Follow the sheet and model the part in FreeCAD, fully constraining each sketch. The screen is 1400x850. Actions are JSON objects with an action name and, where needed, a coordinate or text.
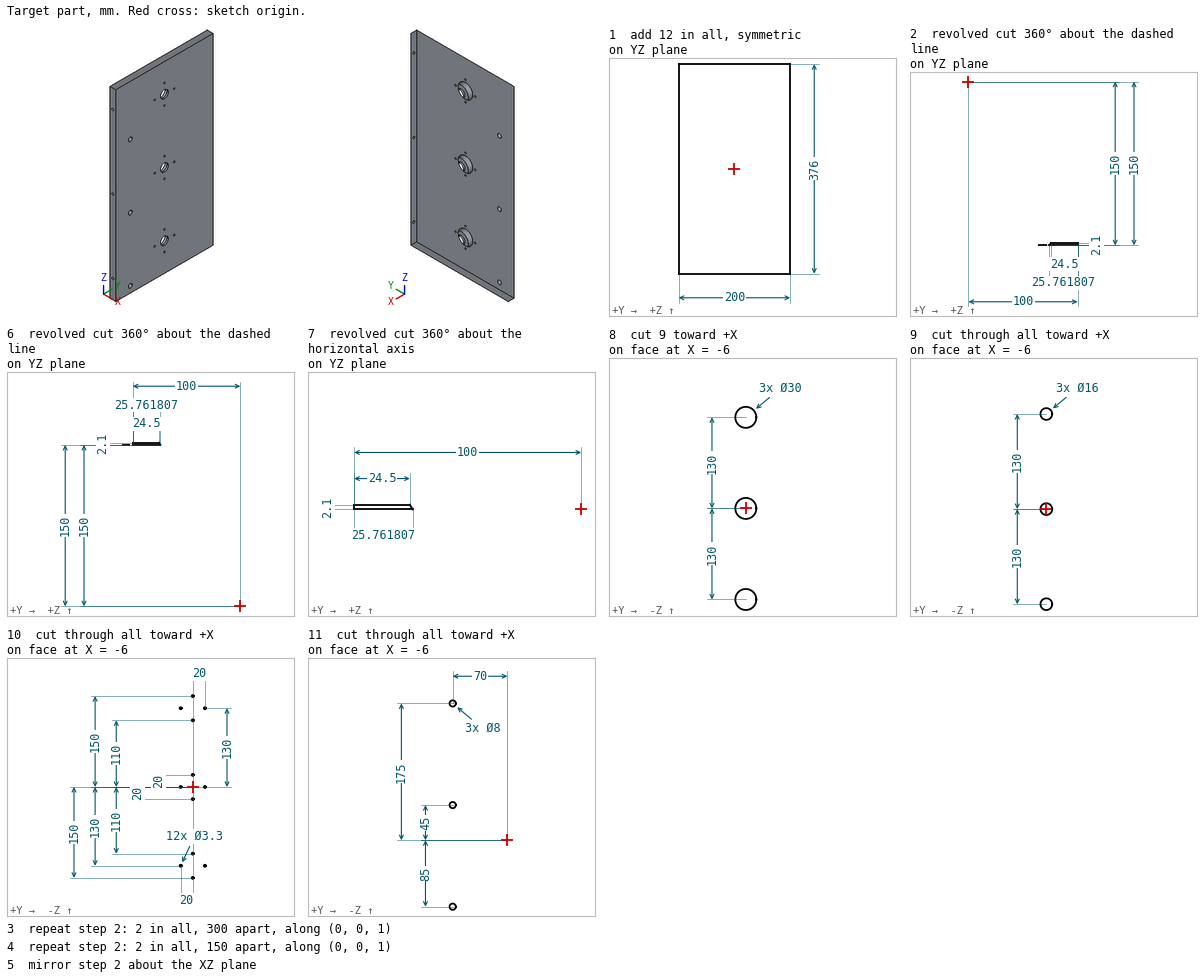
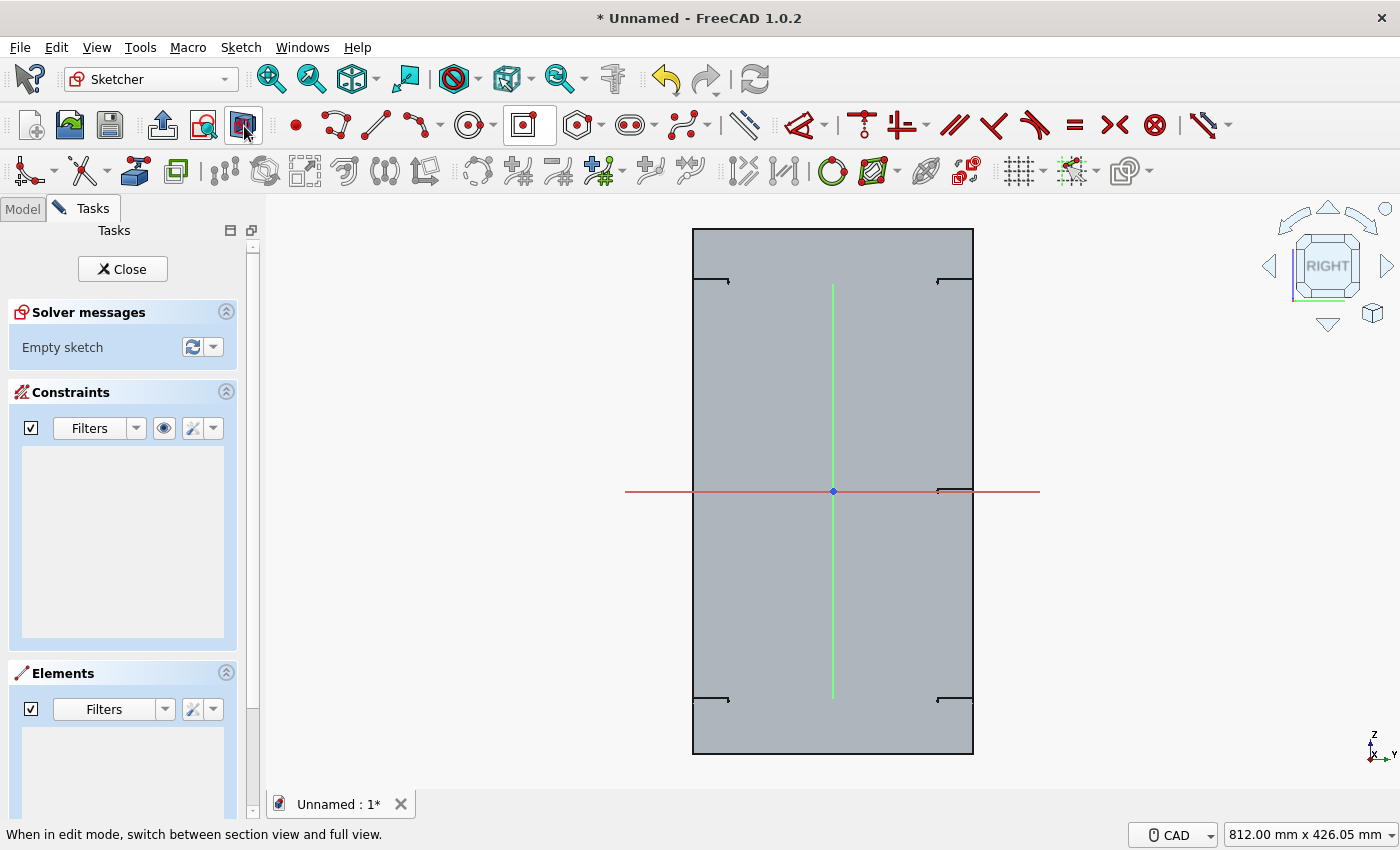
{"action": "scroll", "coordinate": [709, 490], "scroll_direction": "up", "scroll_amount": 15}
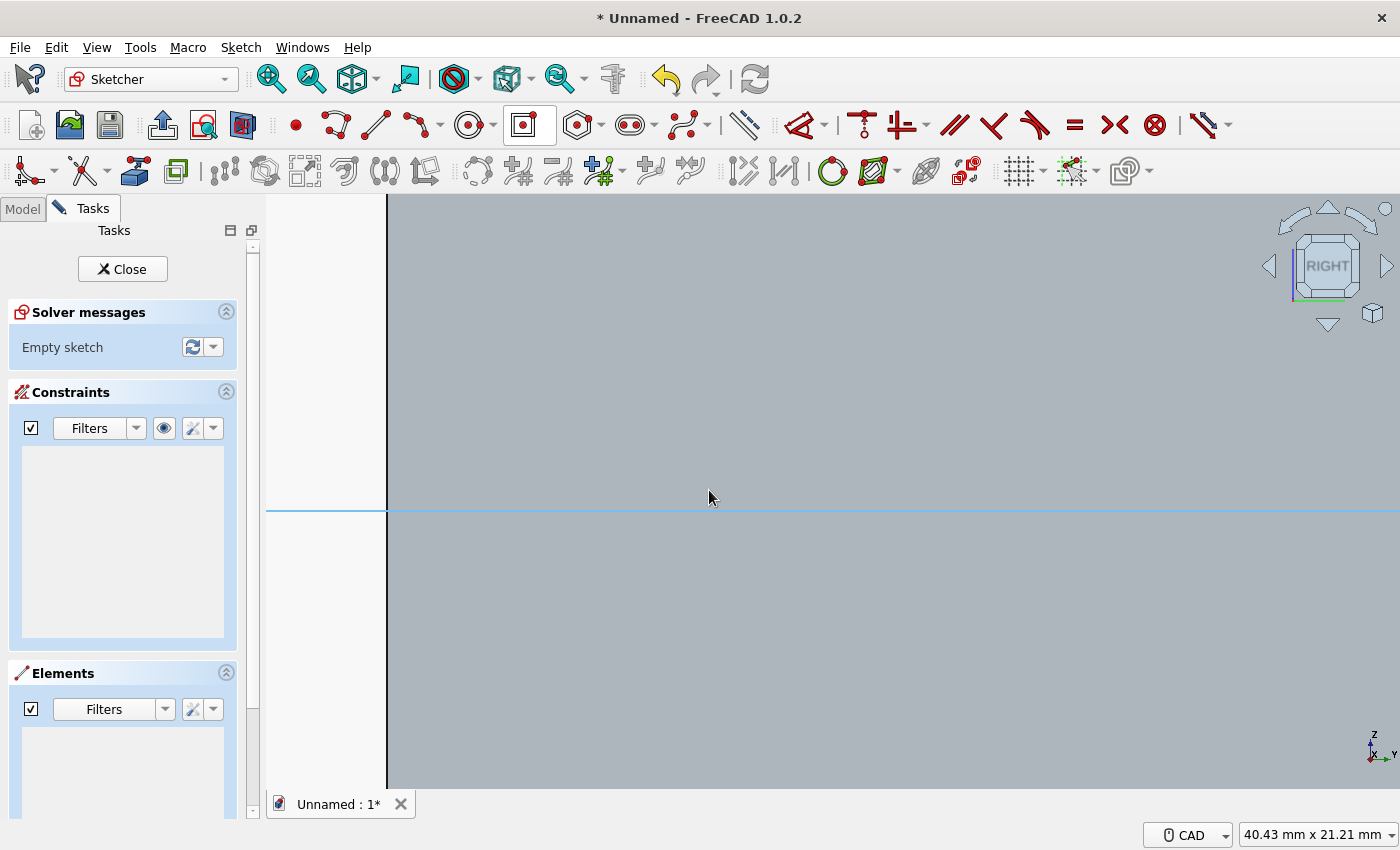
{"action": "left_click", "coordinate": [336, 126]}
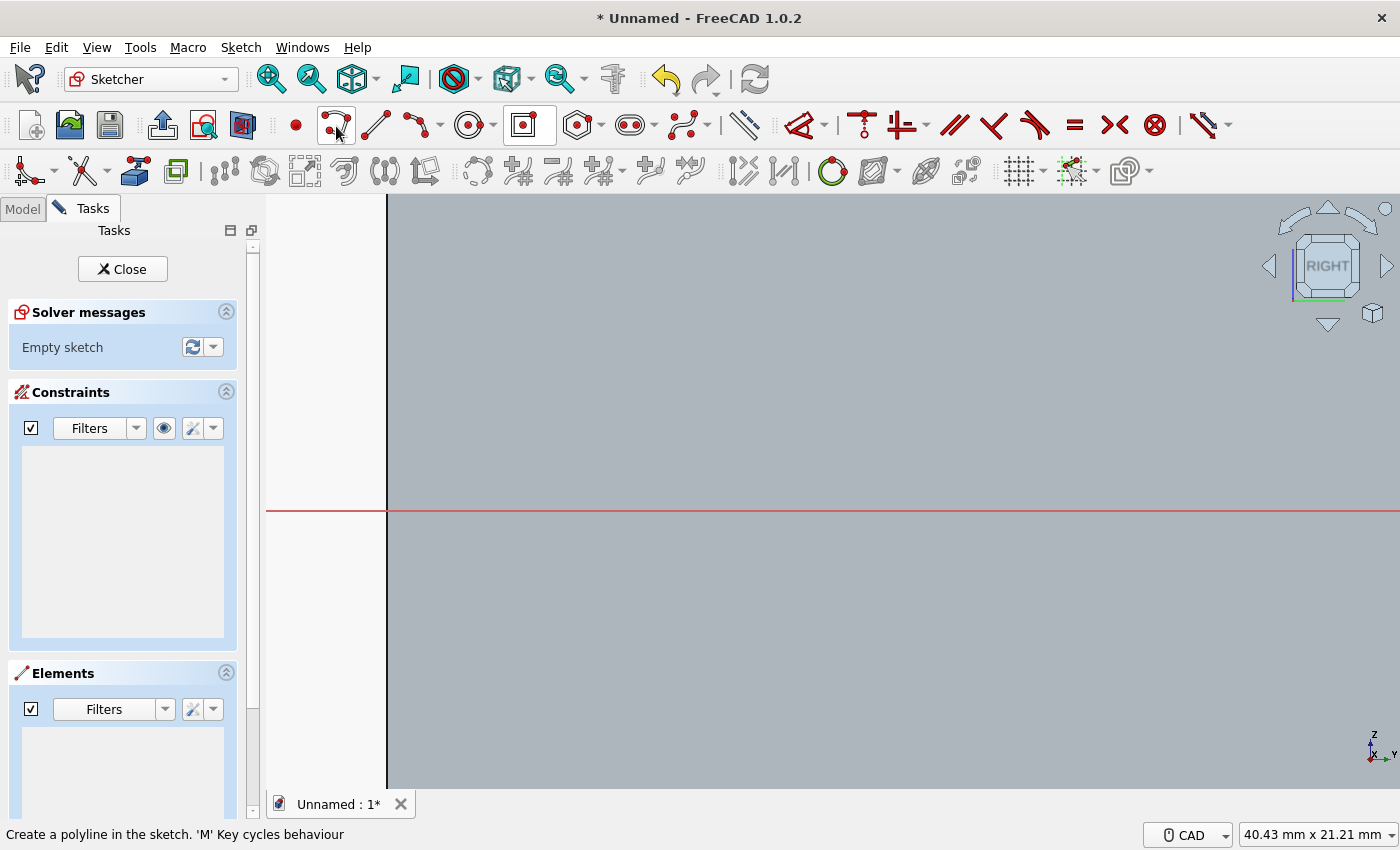
{"action": "left_click", "coordinate": [1110, 511]}
{"action": "left_click", "coordinate": [1074, 452]}
{"action": "left_click", "coordinate": [387, 452]}
{"action": "left_click", "coordinate": [387, 502]}
{"action": "left_click", "coordinate": [1110, 511]}
{"action": "key", "text": "Escape"}
{"action": "key", "text": "Escape"}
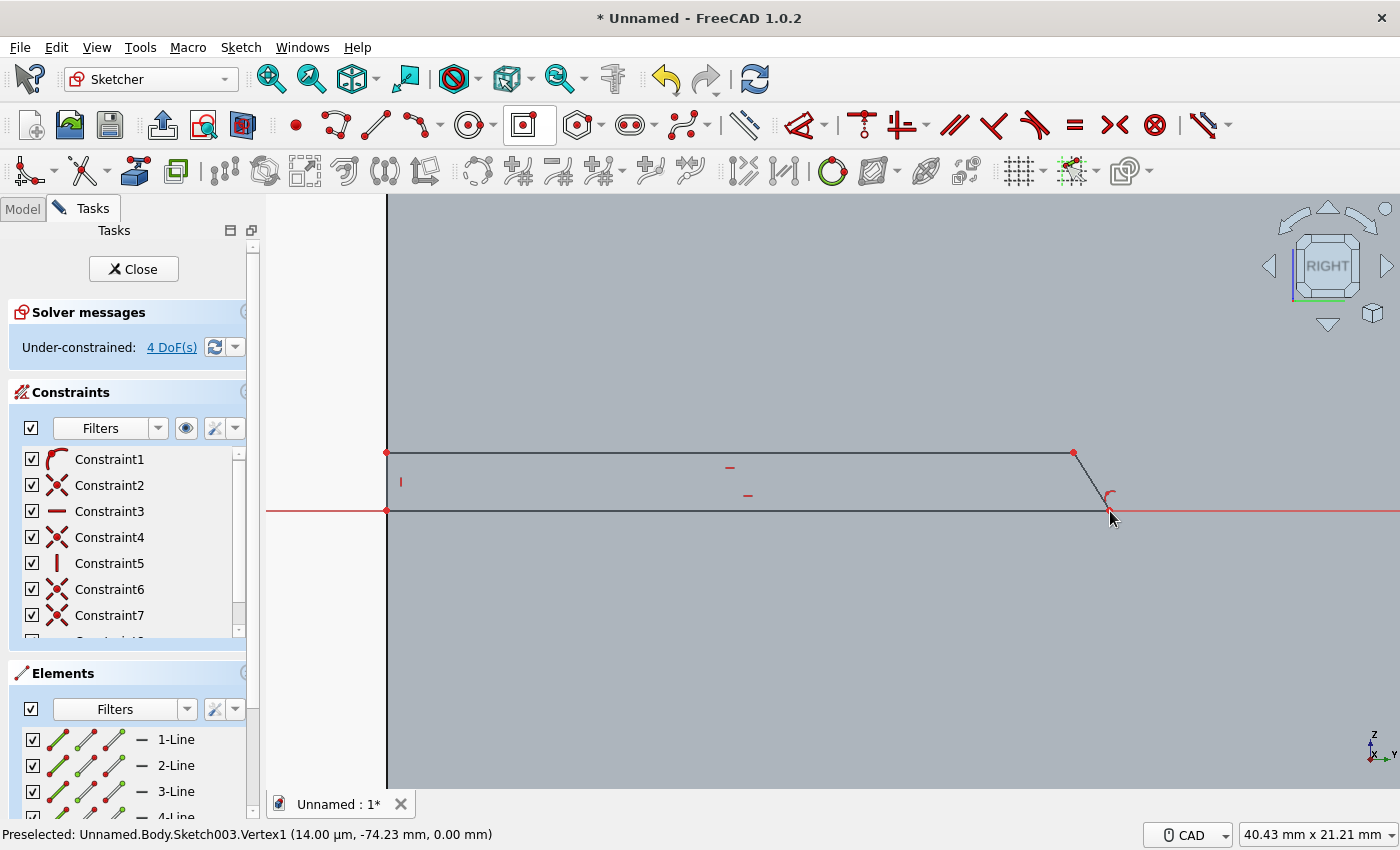
{"action": "left_click", "coordinate": [800, 126]}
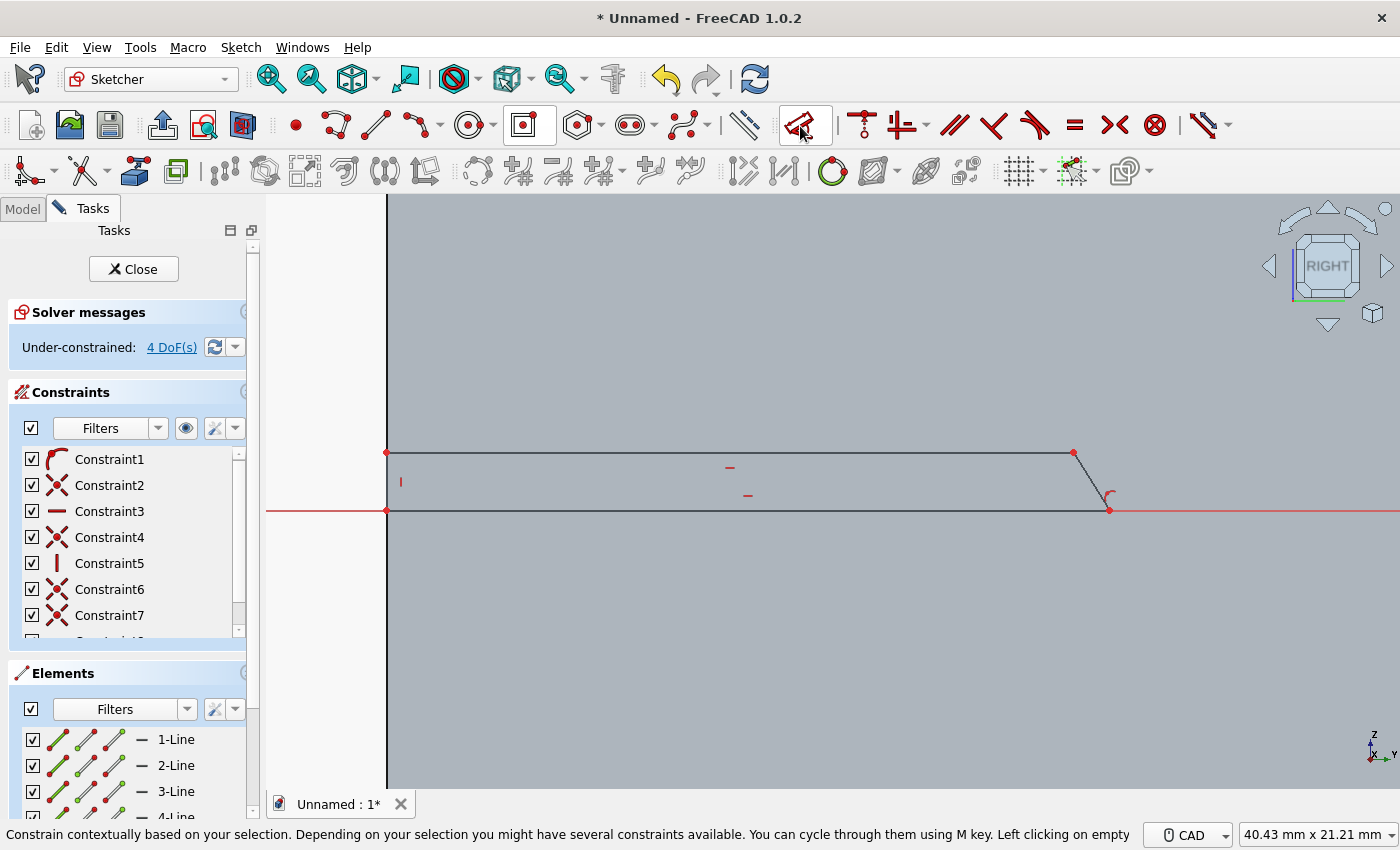
{"action": "left_click", "coordinate": [387, 470]}
{"action": "left_click", "coordinate": [353, 482]}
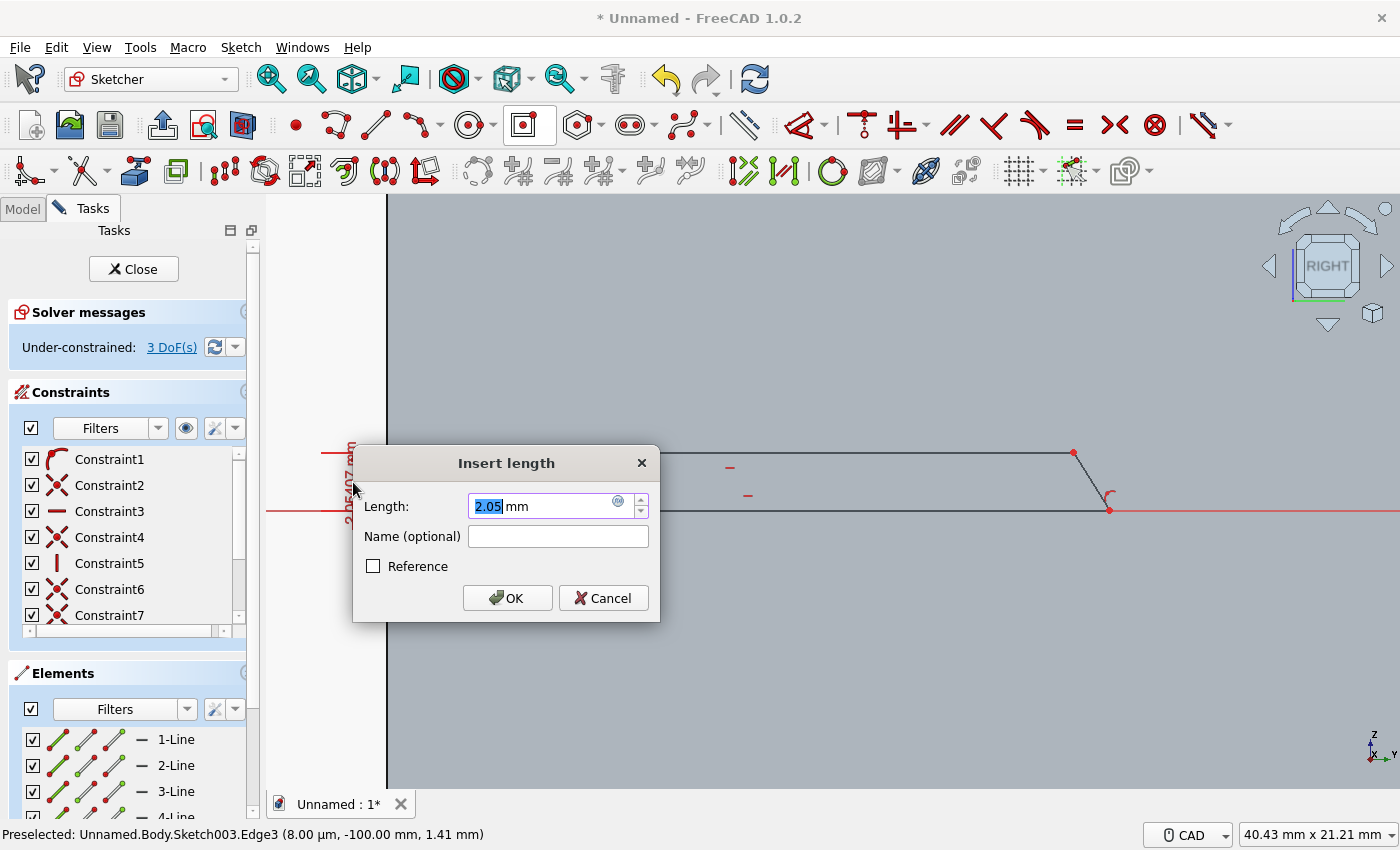
{"action": "type", "text": "2.1"}
{"action": "key", "text": "Return"}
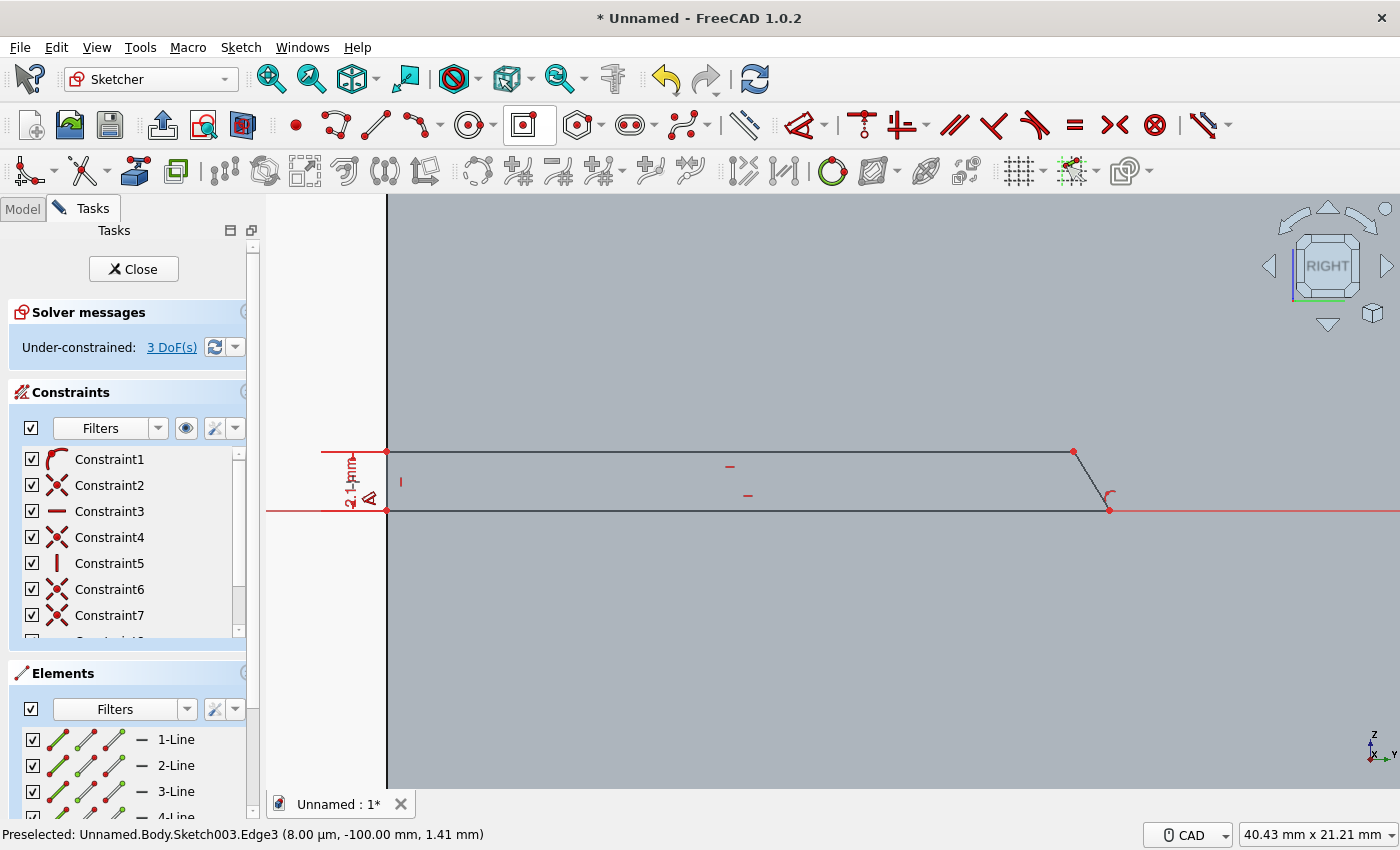
{"action": "left_click", "coordinate": [868, 452]}
{"action": "left_click", "coordinate": [730, 418]}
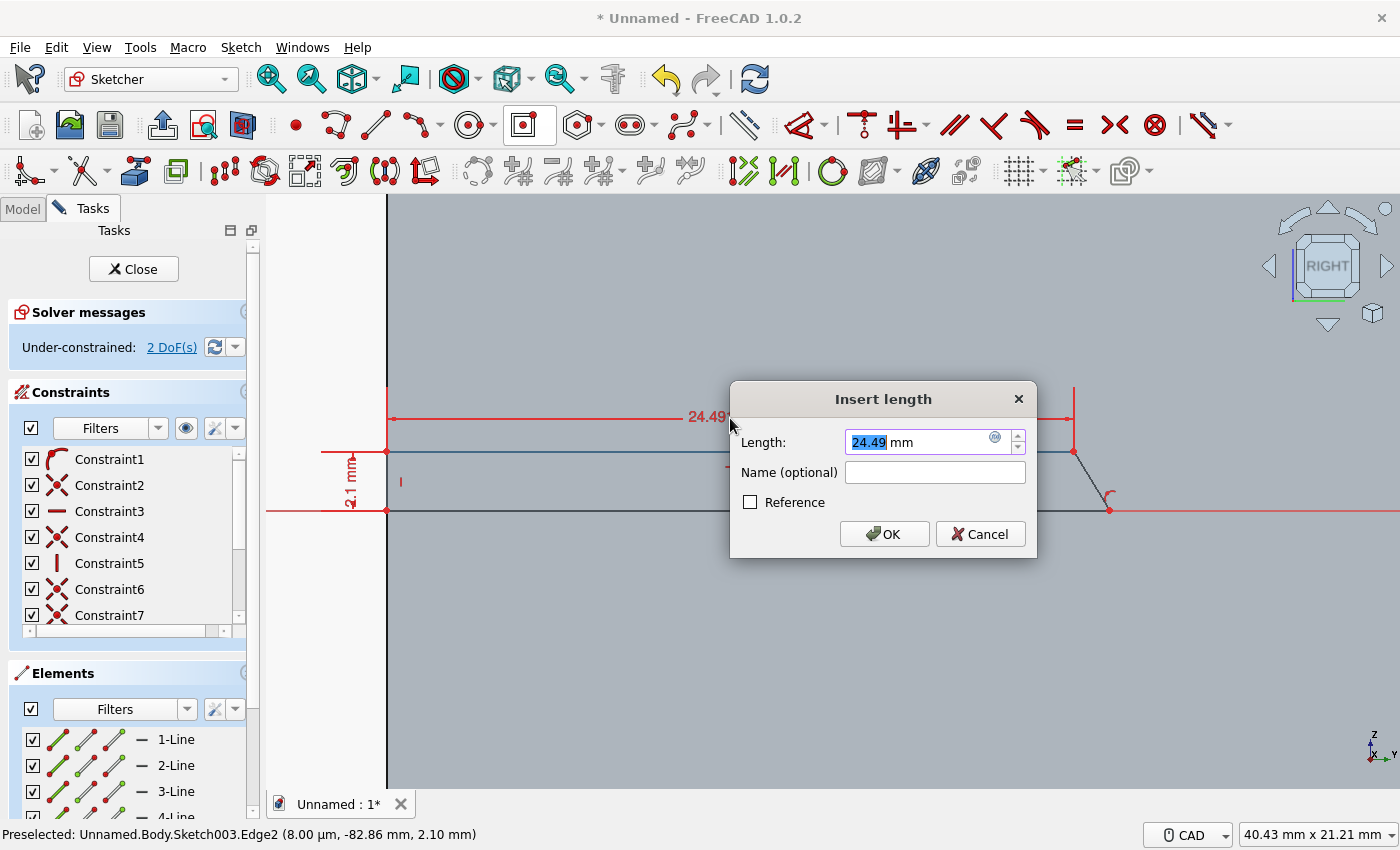
{"action": "type", "text": "24.5"}
{"action": "key", "text": "Return"}